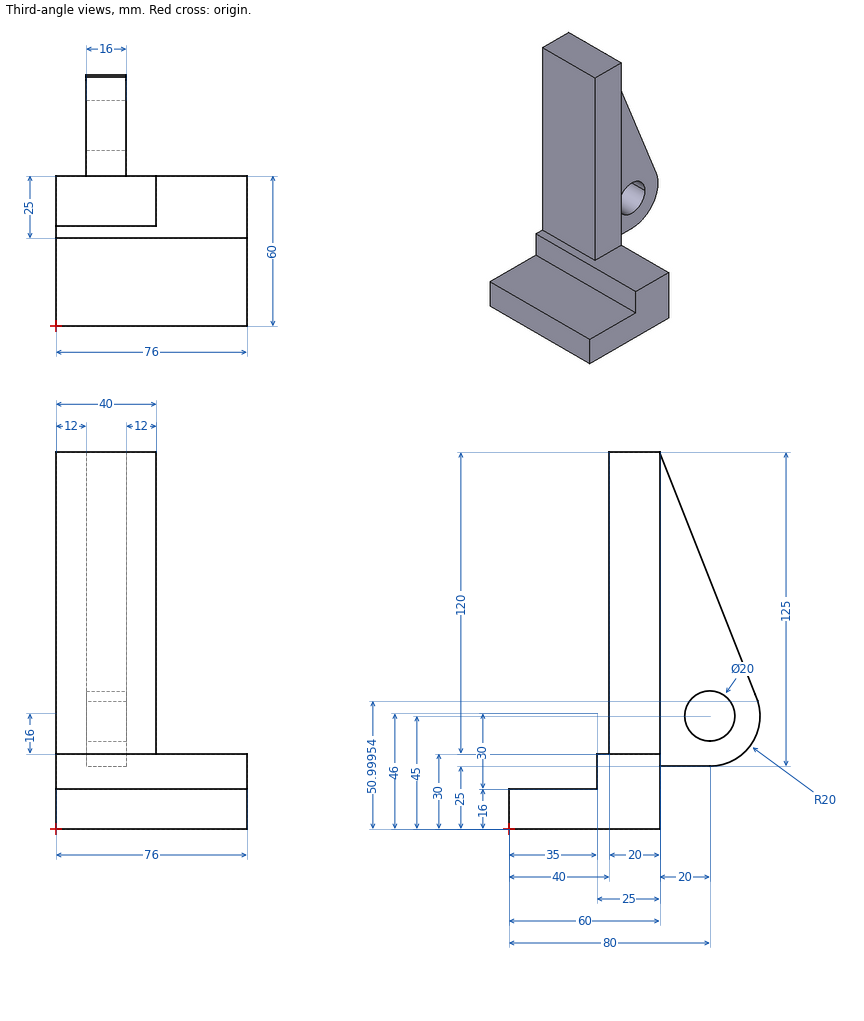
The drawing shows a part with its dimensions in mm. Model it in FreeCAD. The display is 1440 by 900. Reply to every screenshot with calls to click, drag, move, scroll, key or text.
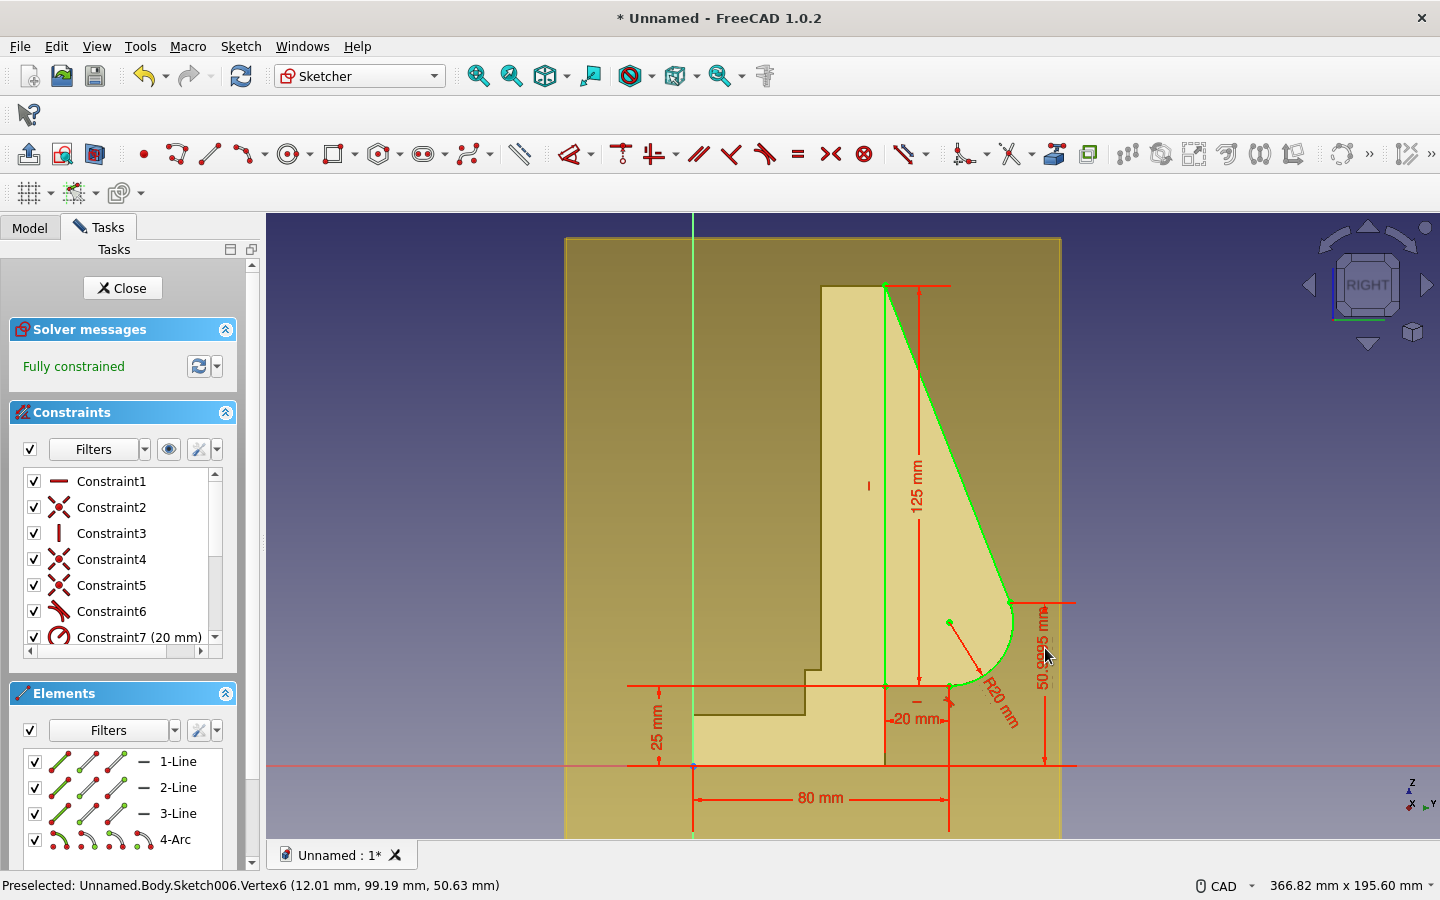
click(123, 288)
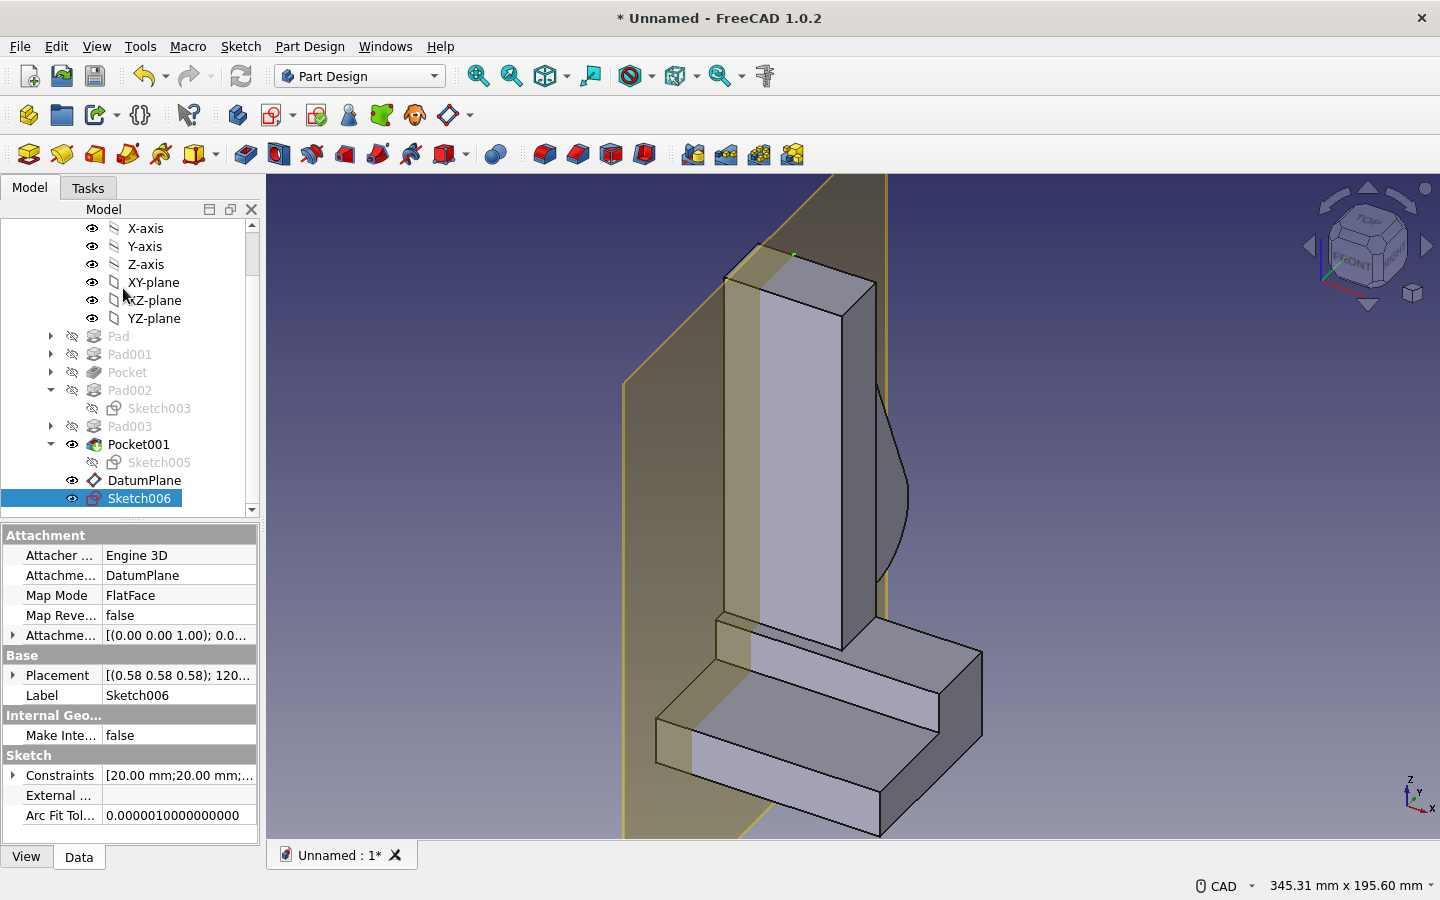
click(246, 154)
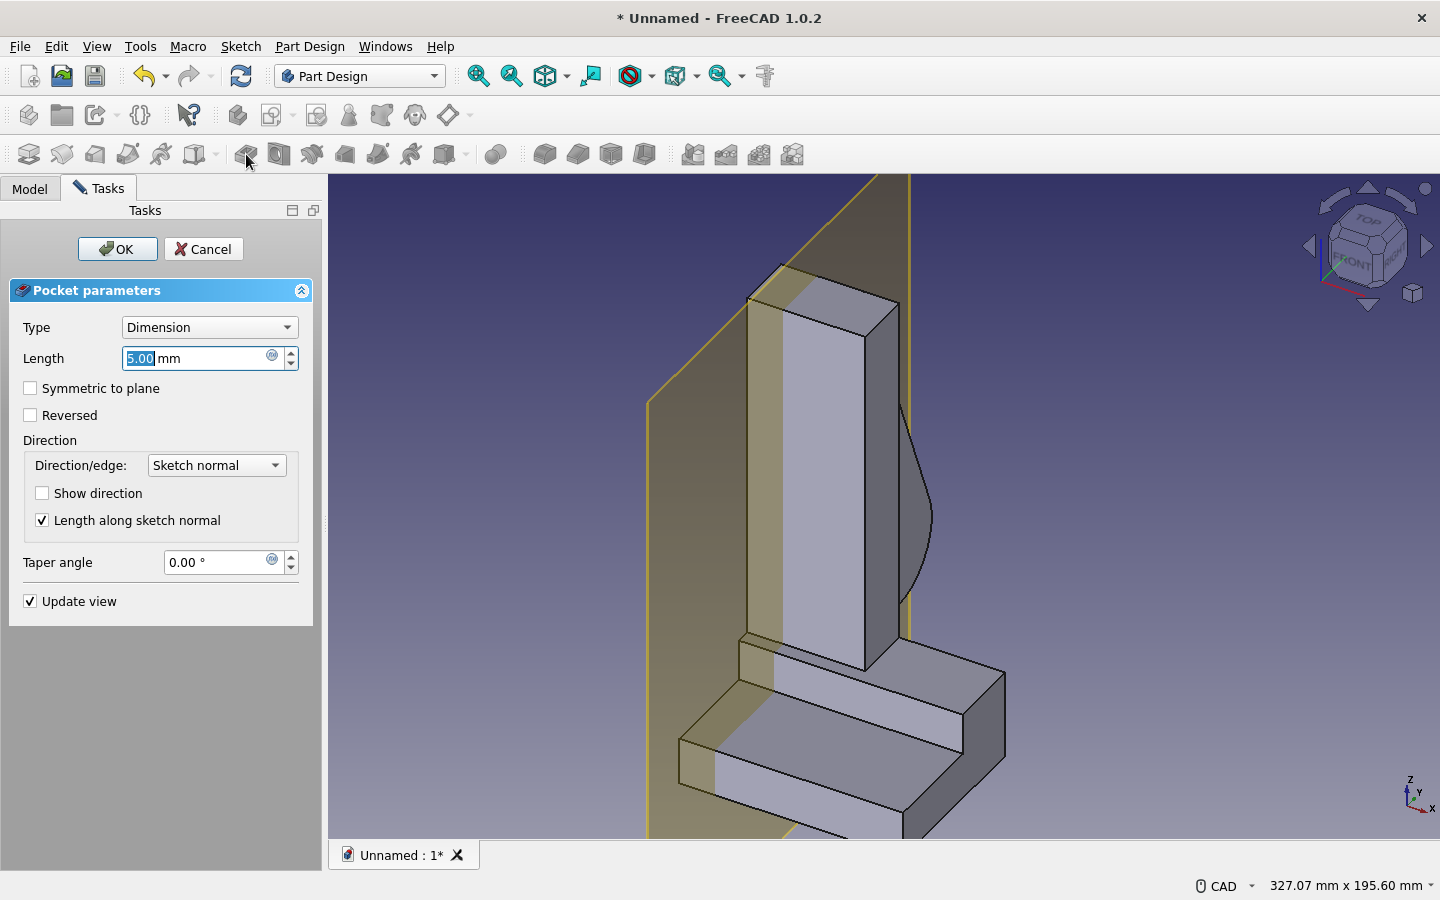
text(12)
key(Tab)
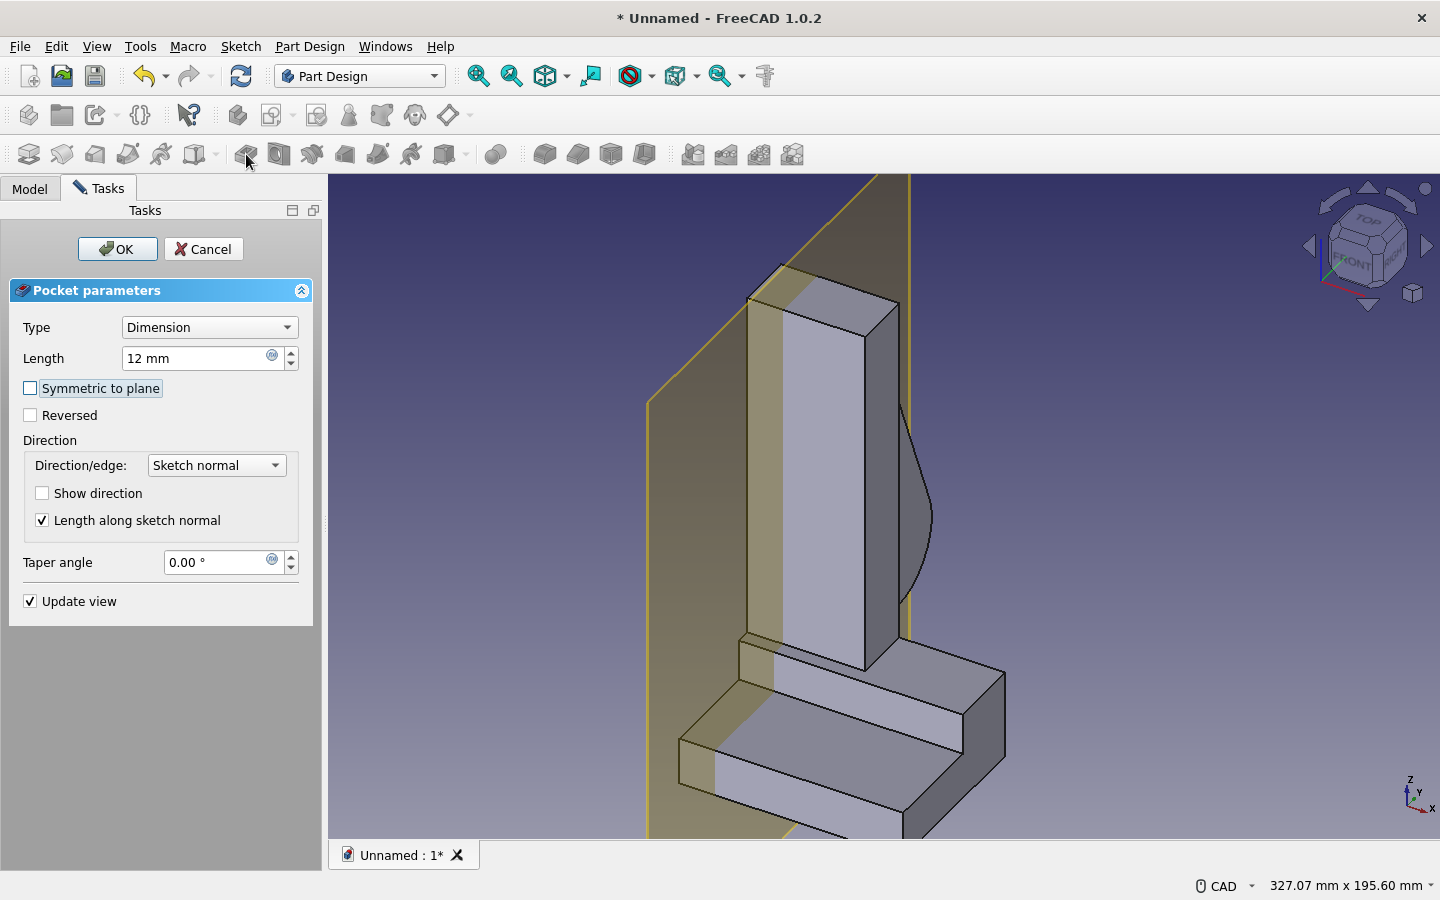
click(118, 249)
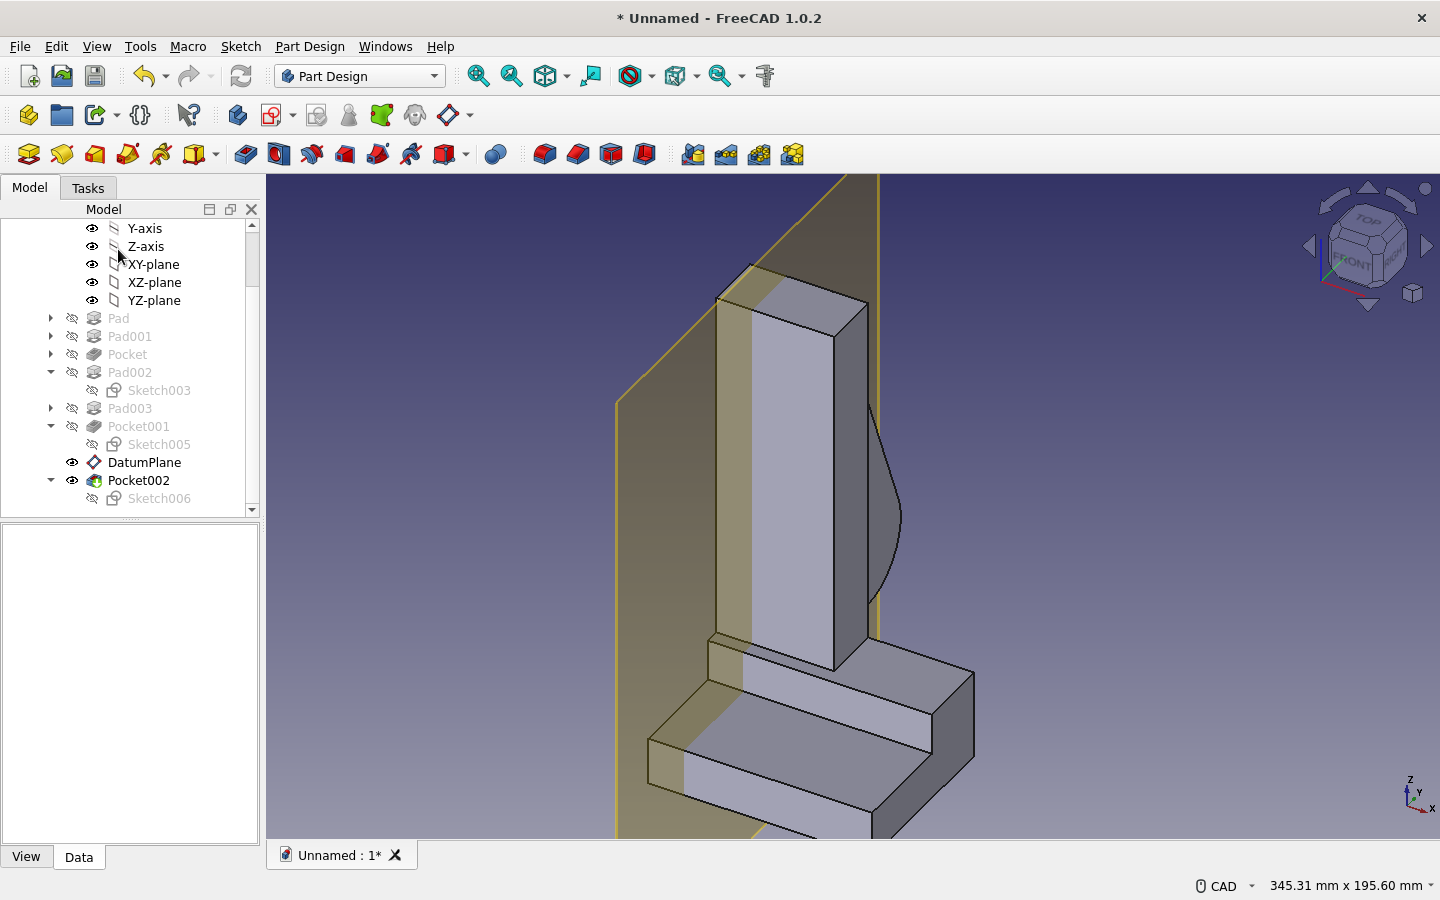
click(117, 462)
key(space)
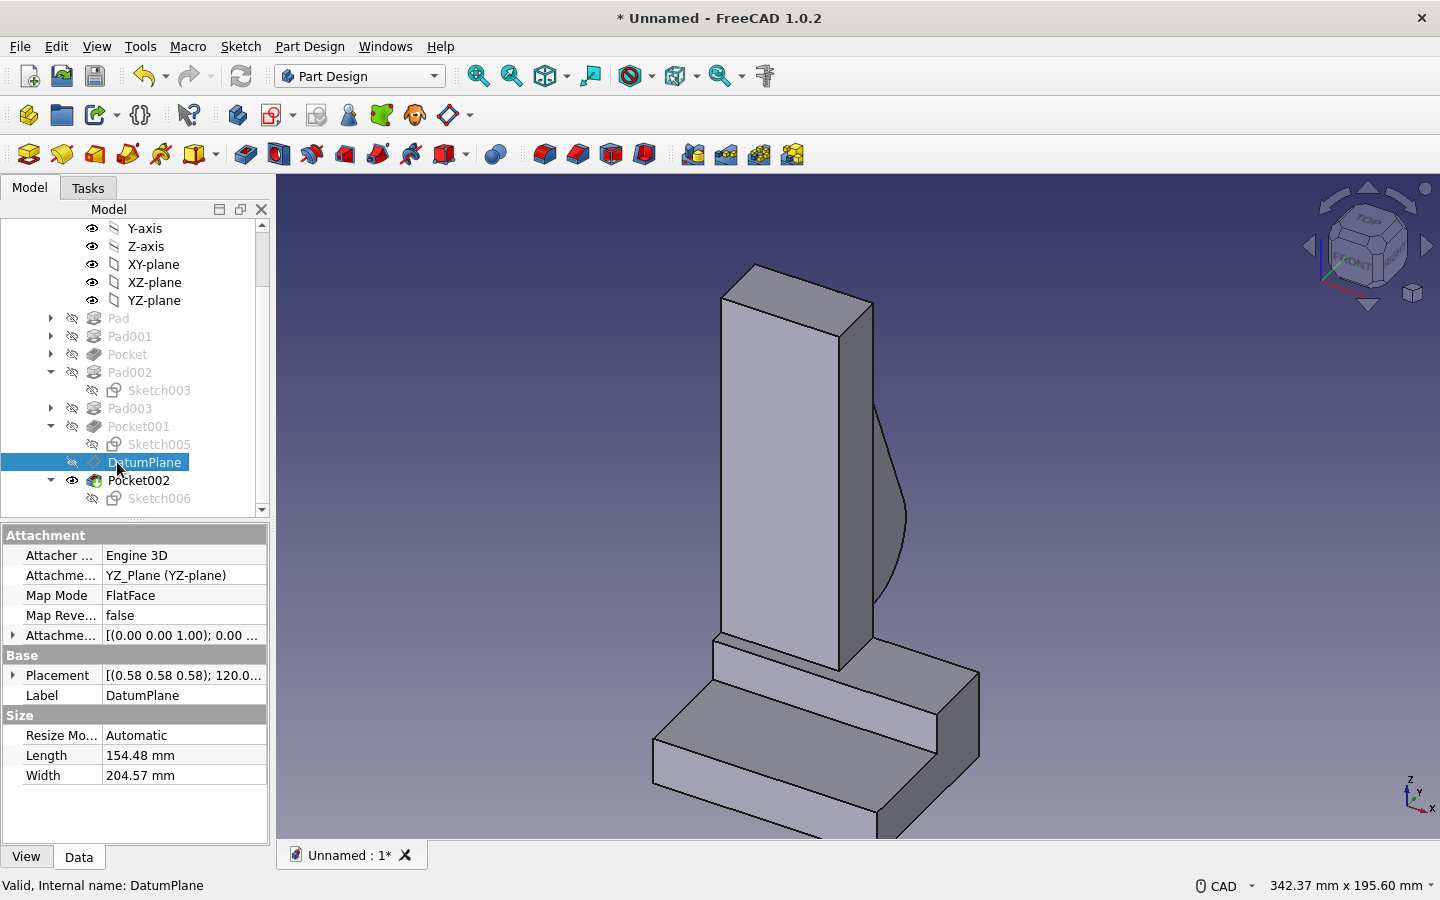
key(v)
key(f)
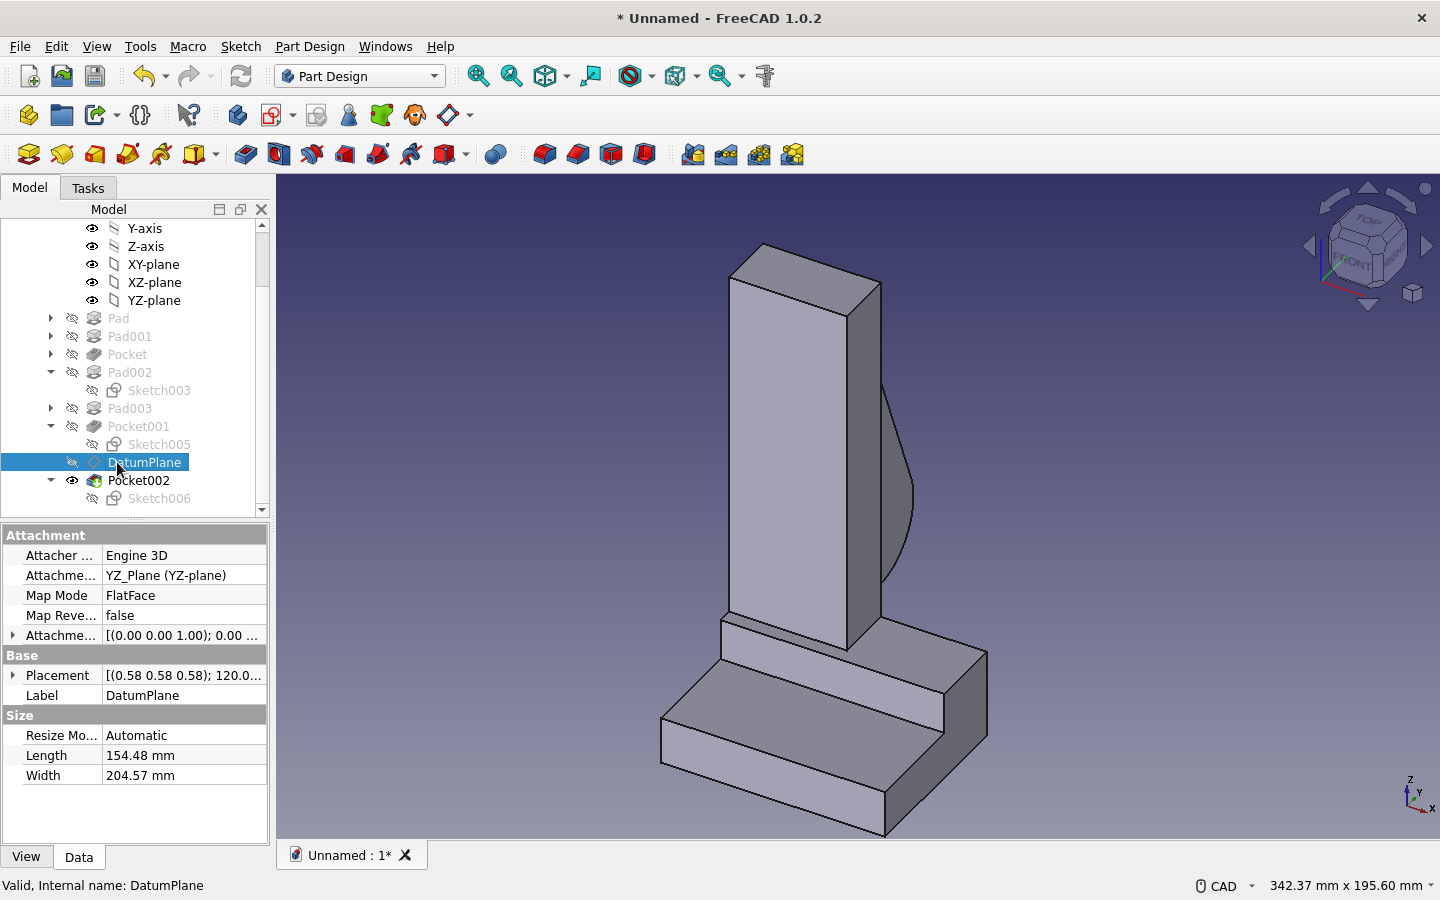
click(889, 500)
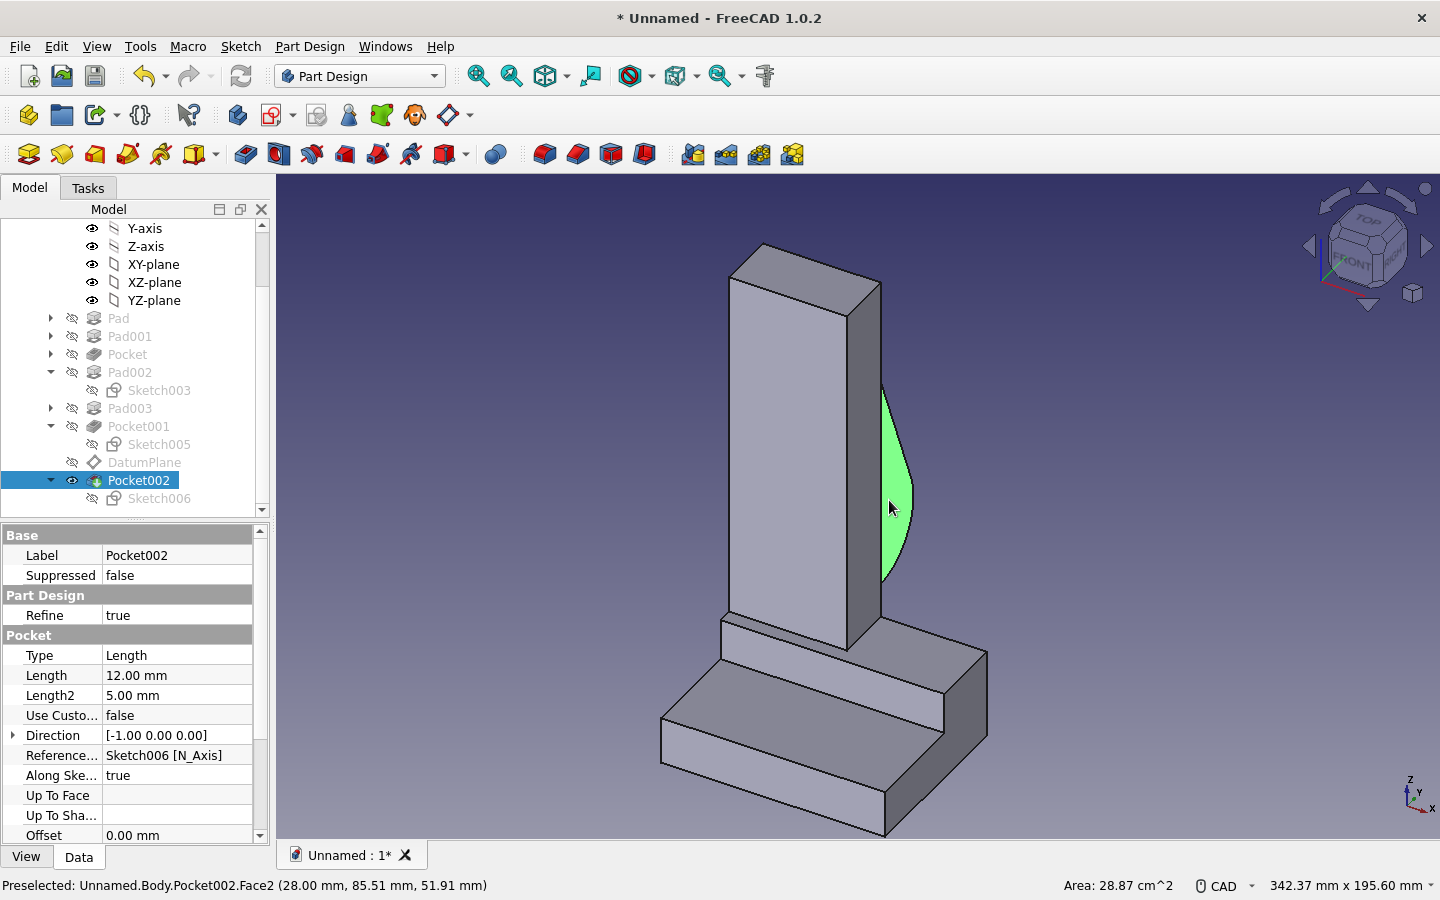
click(270, 116)